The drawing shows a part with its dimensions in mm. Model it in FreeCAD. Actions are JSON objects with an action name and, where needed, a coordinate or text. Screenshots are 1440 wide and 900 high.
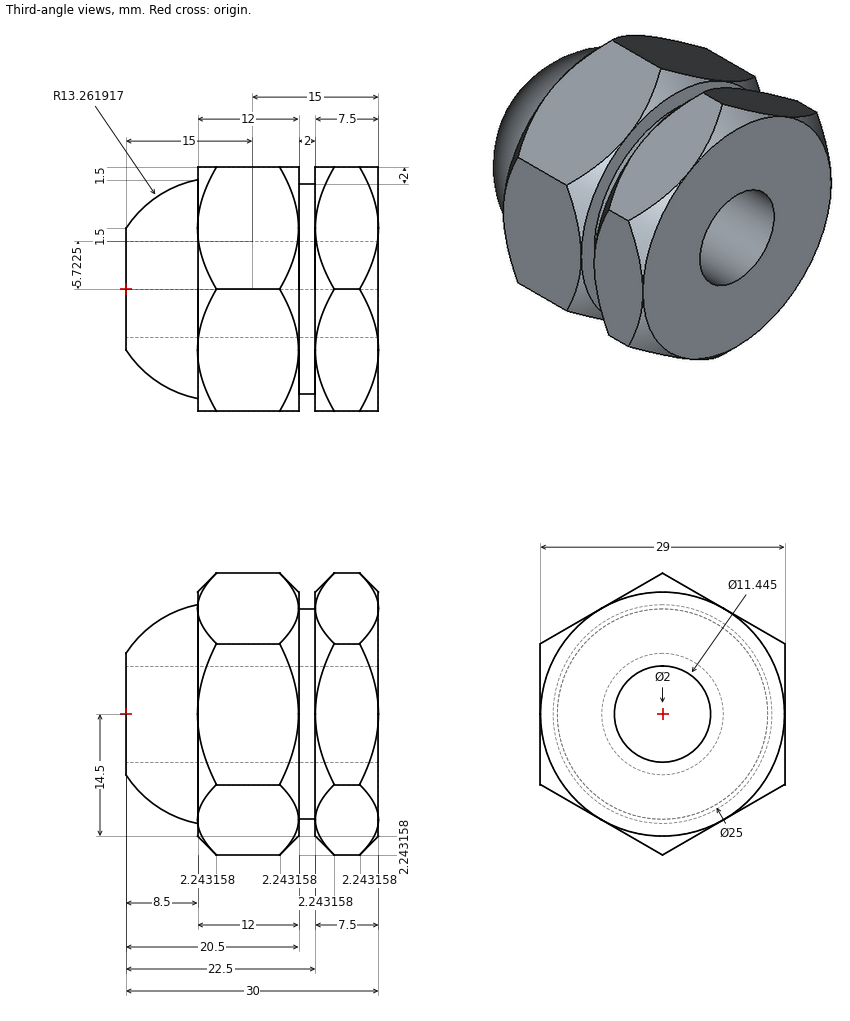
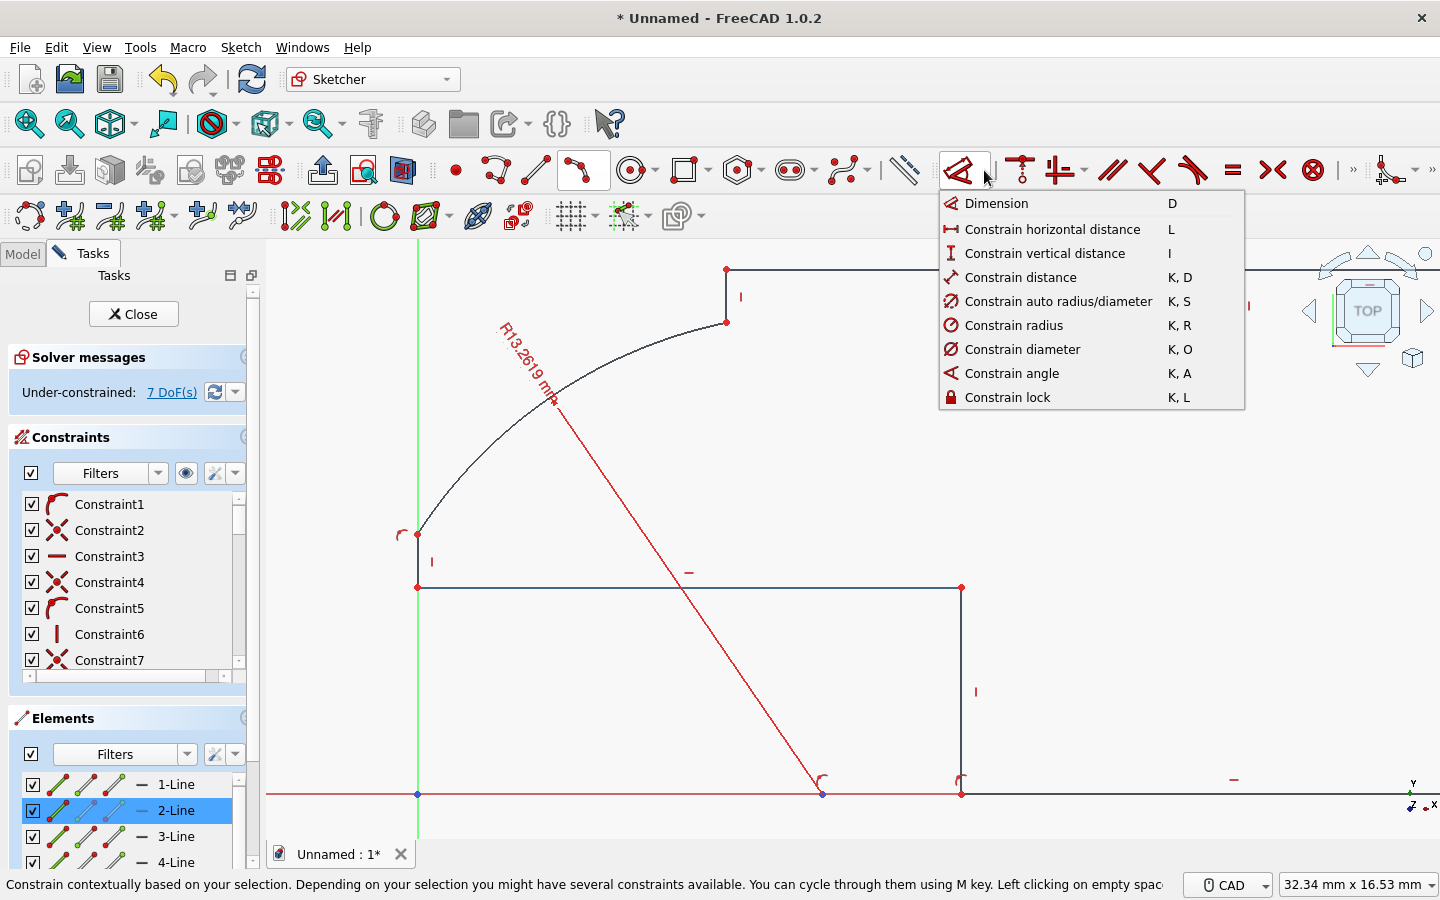
{"action": "left_click", "coordinate": [1092, 229]}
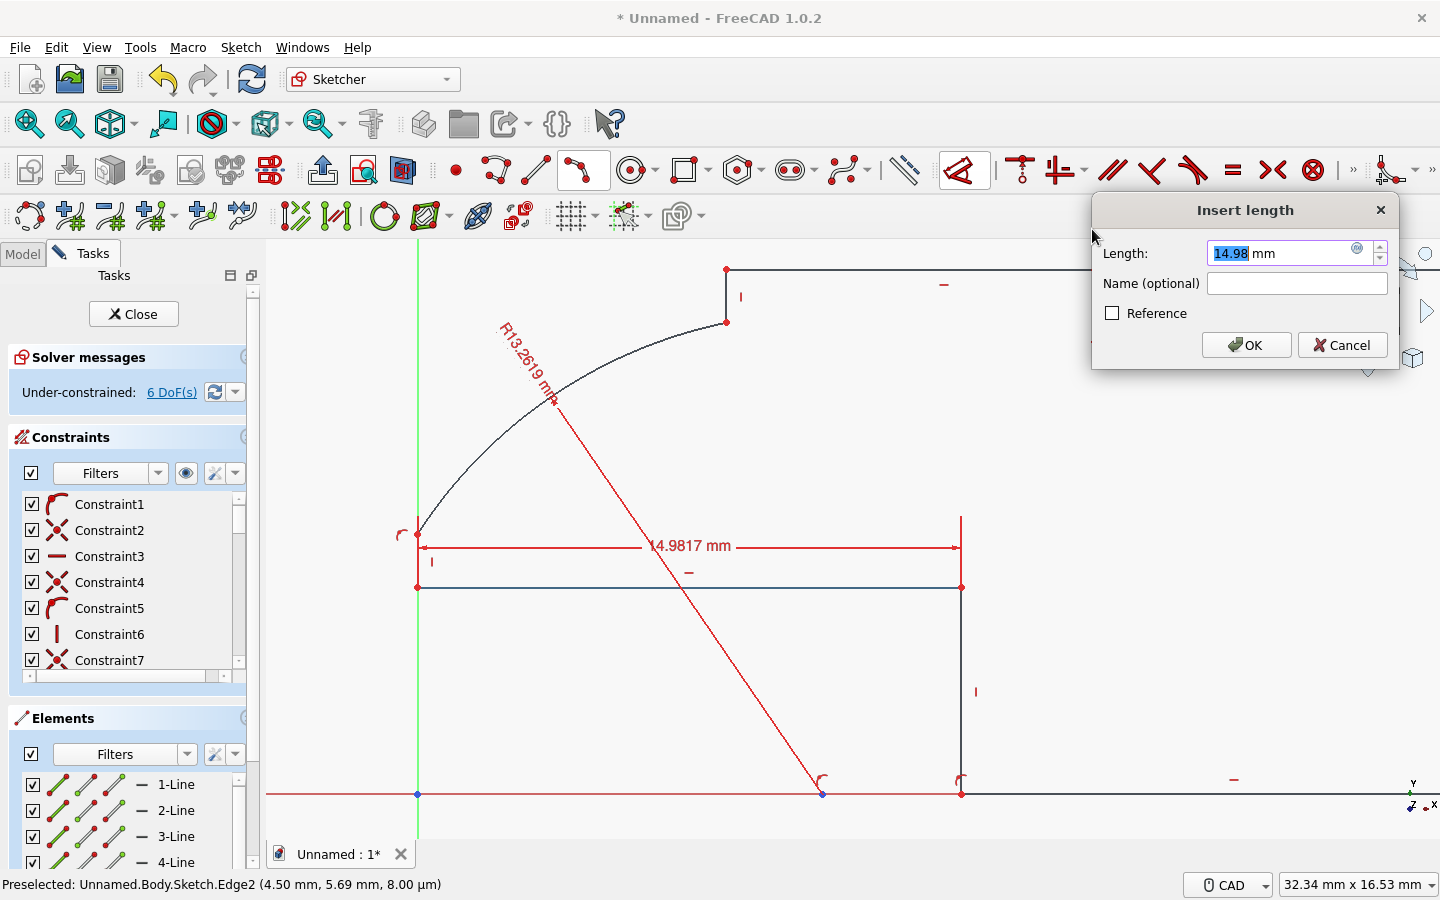
{"action": "type", "text": "15"}
{"action": "key", "text": "Return"}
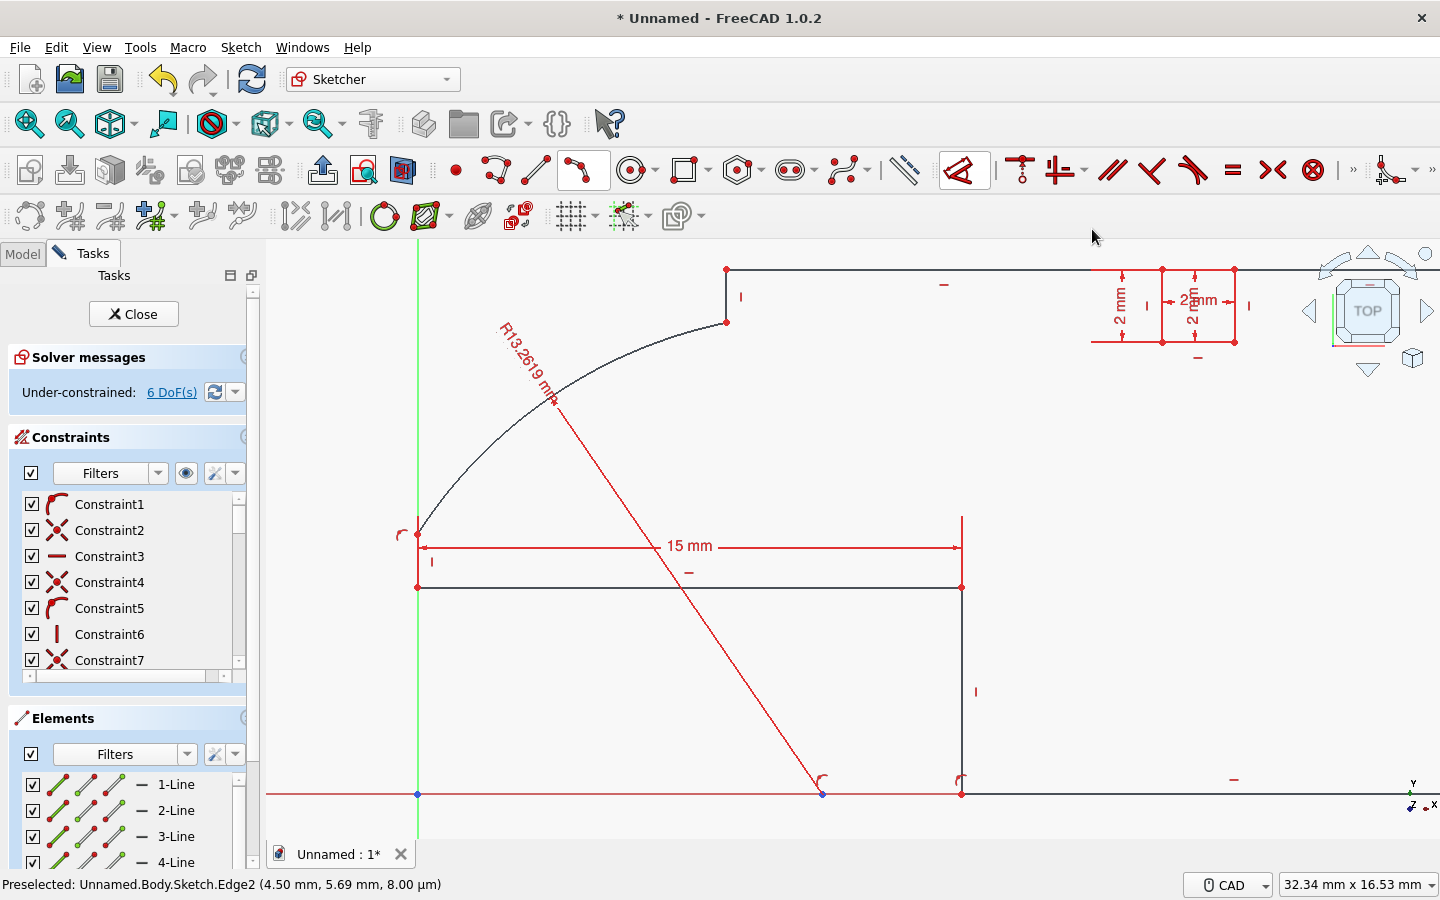
{"action": "left_click", "coordinate": [1125, 794]}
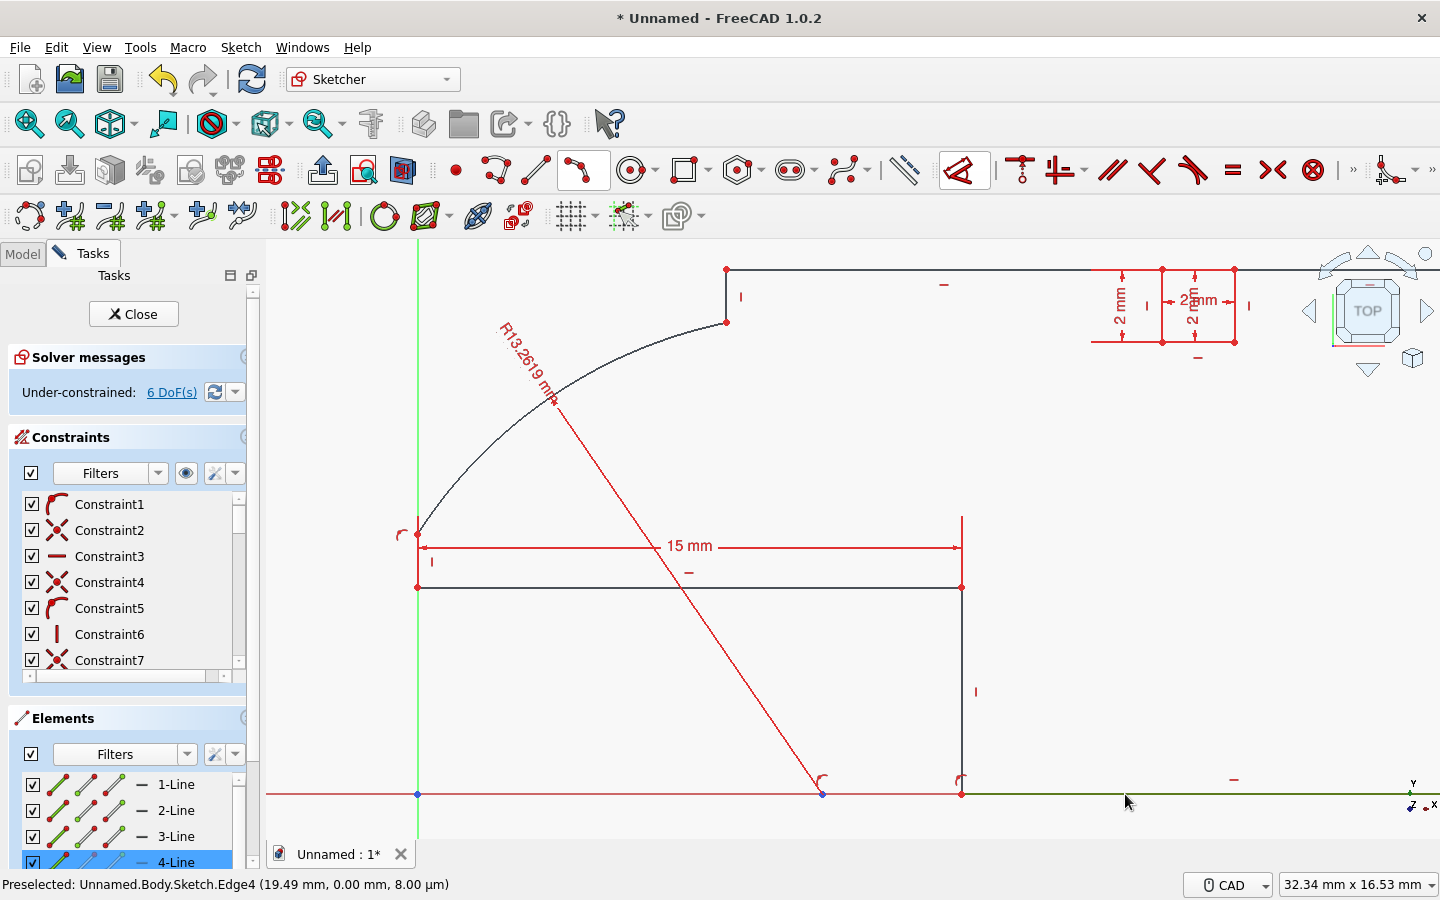
{"action": "left_click", "coordinate": [984, 170]}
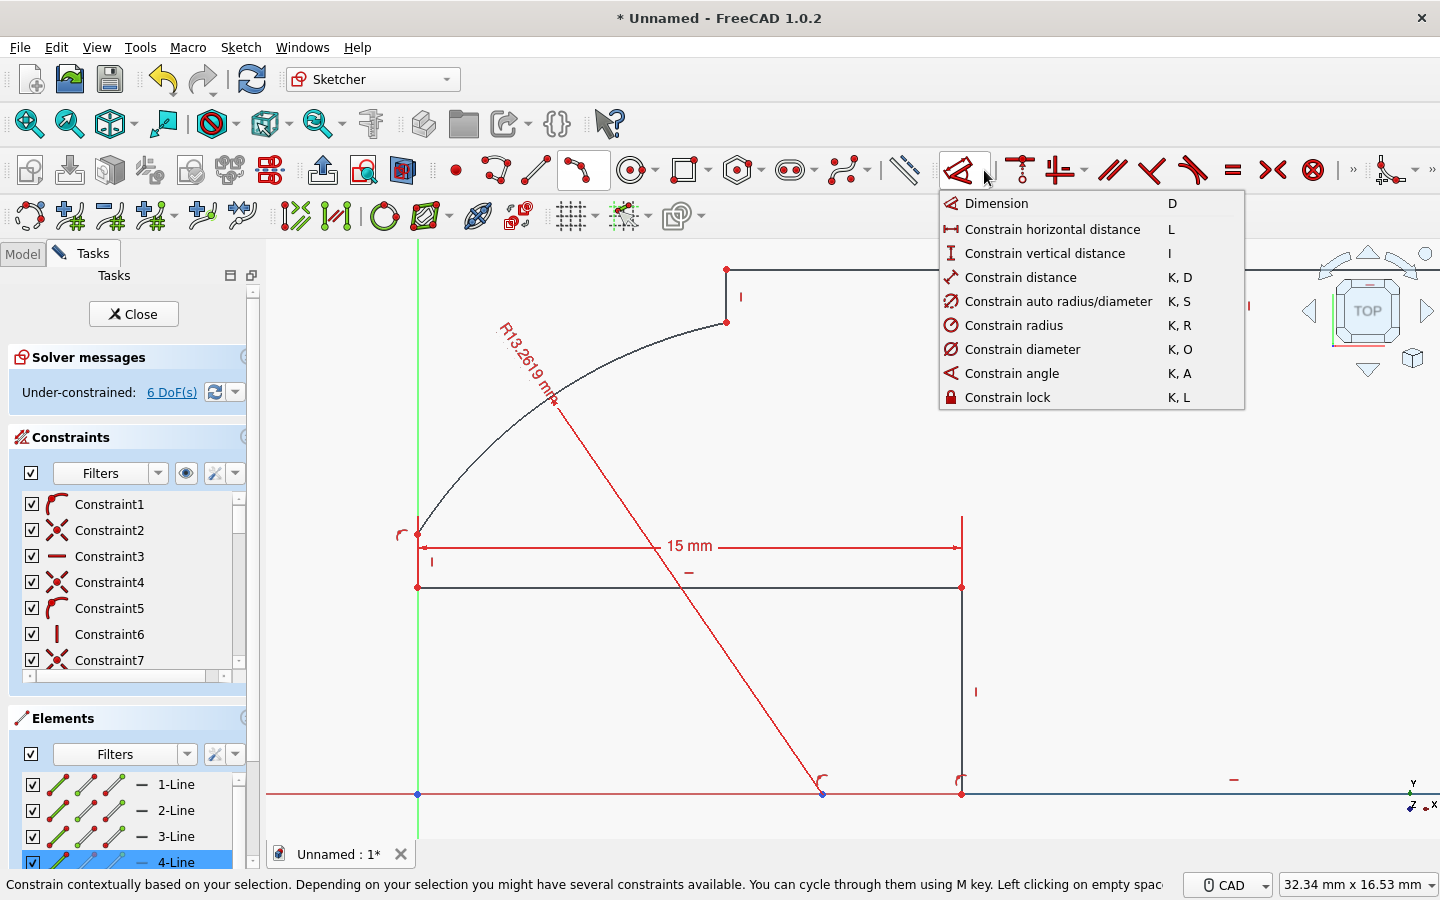
{"action": "left_click", "coordinate": [1092, 229]}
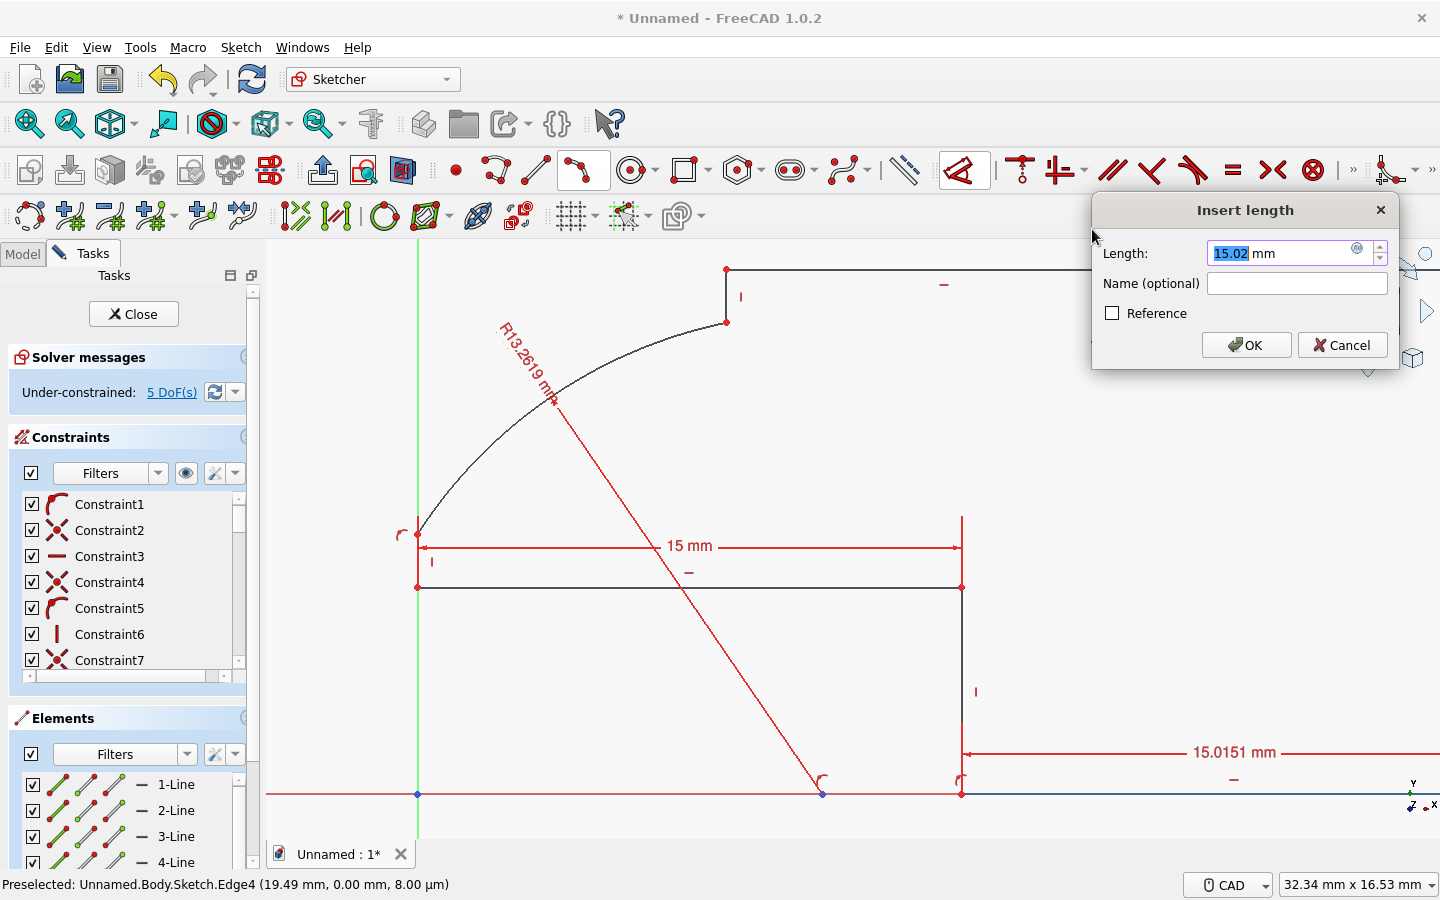
{"action": "type", "text": "15"}
{"action": "key", "text": "Return"}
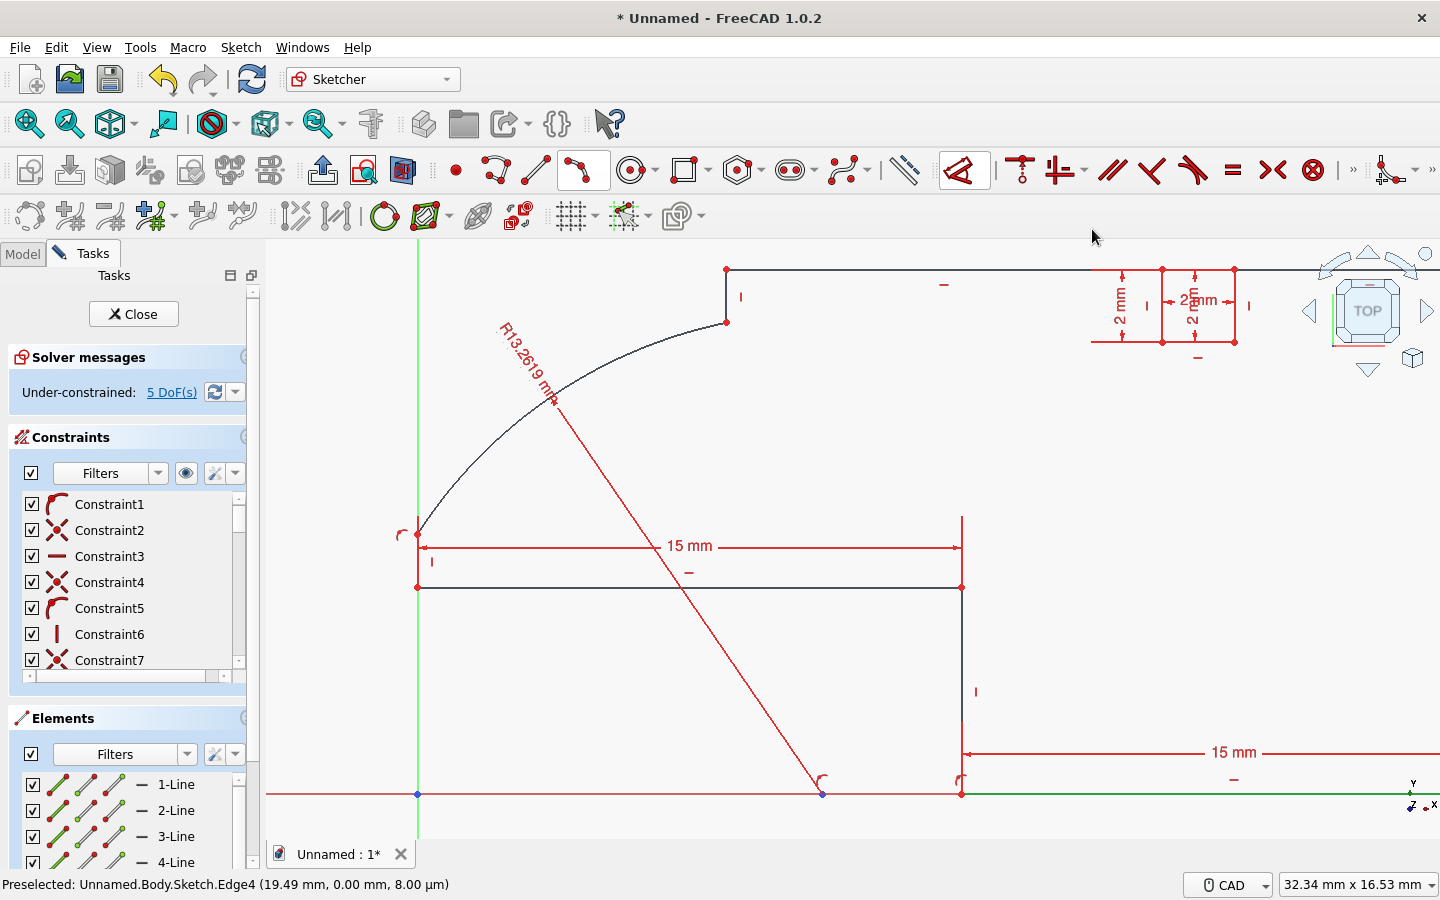
{"action": "left_click", "coordinate": [1032, 270]}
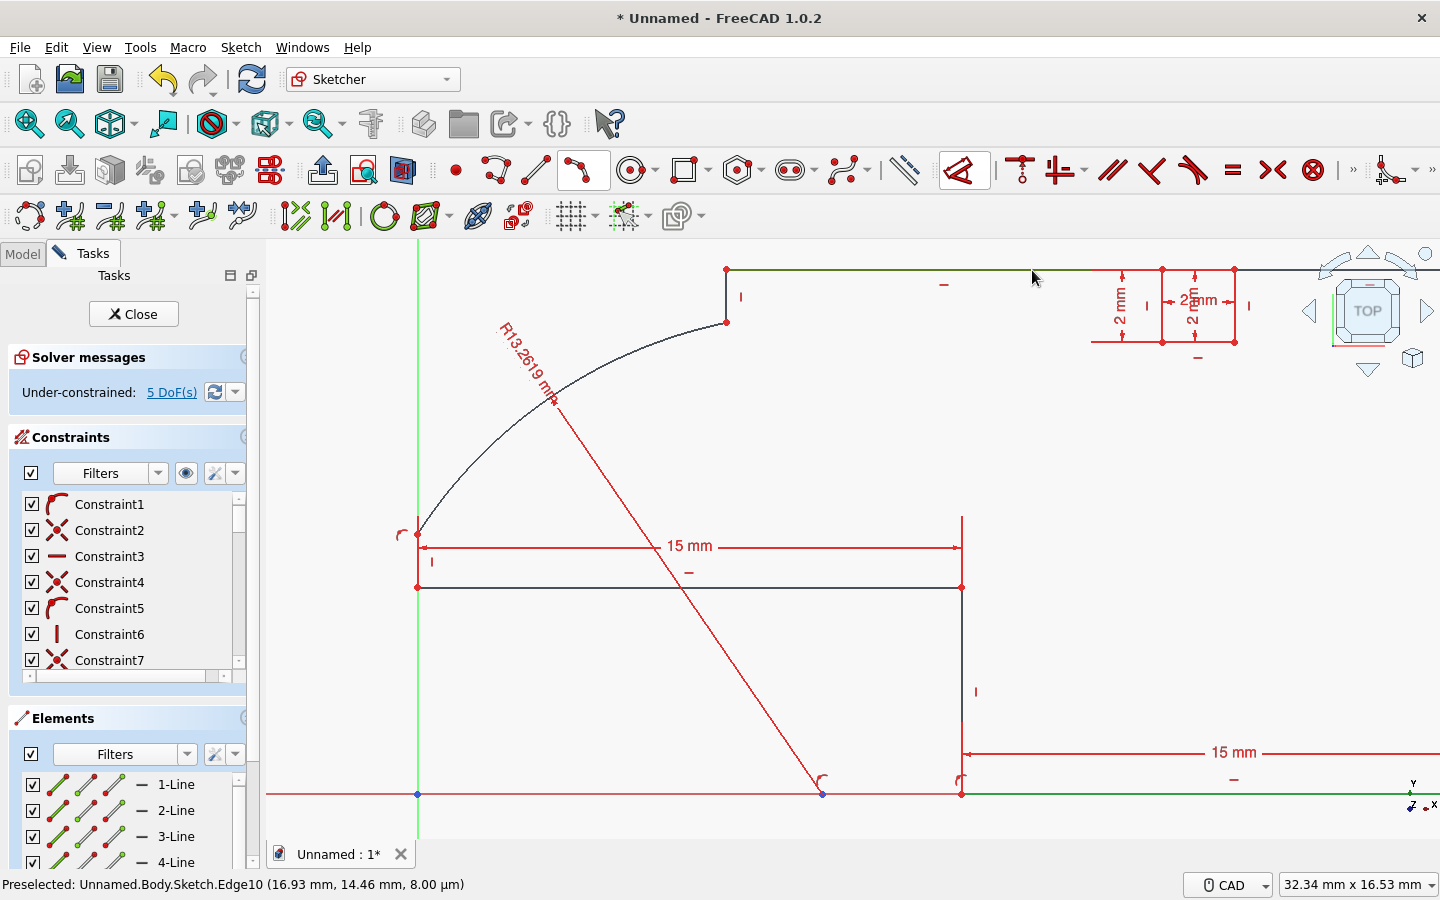
{"action": "left_click", "coordinate": [984, 170]}